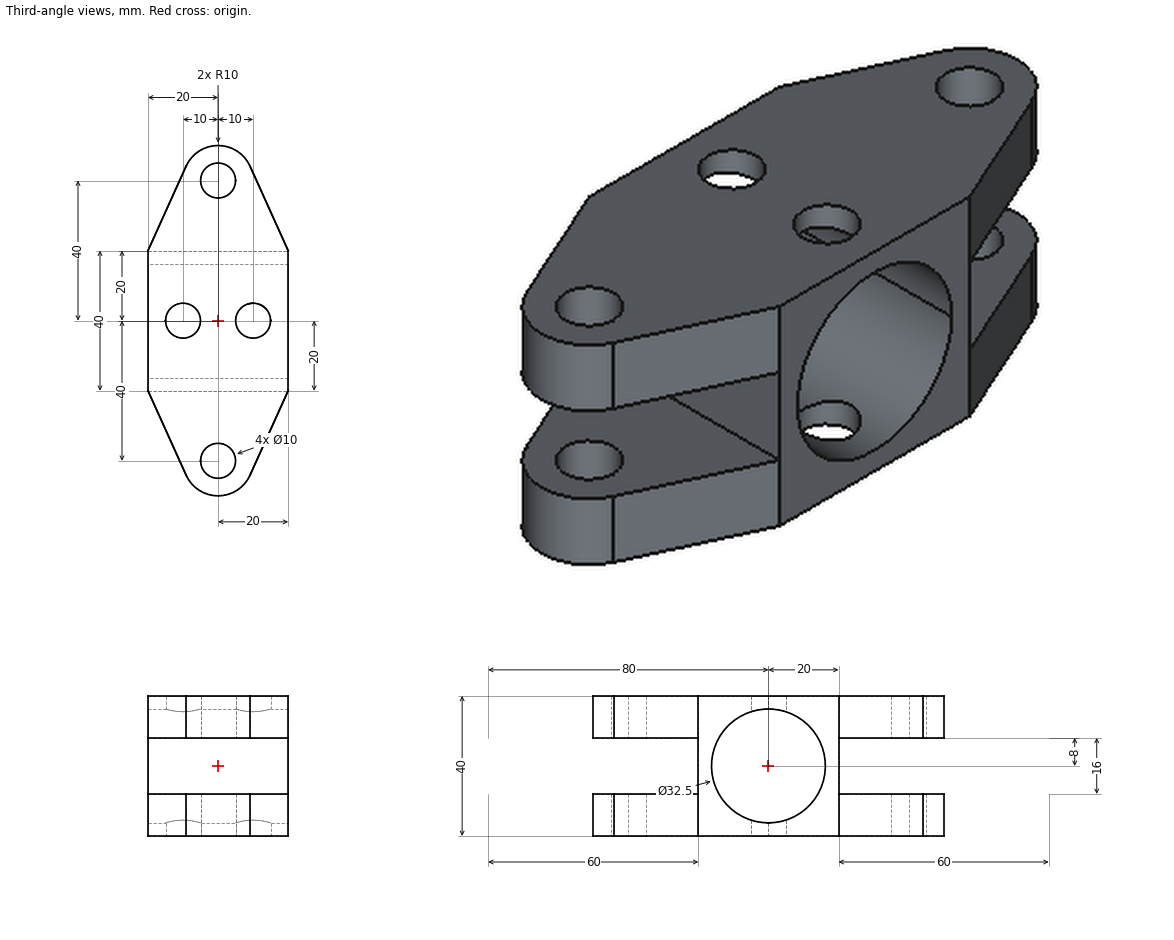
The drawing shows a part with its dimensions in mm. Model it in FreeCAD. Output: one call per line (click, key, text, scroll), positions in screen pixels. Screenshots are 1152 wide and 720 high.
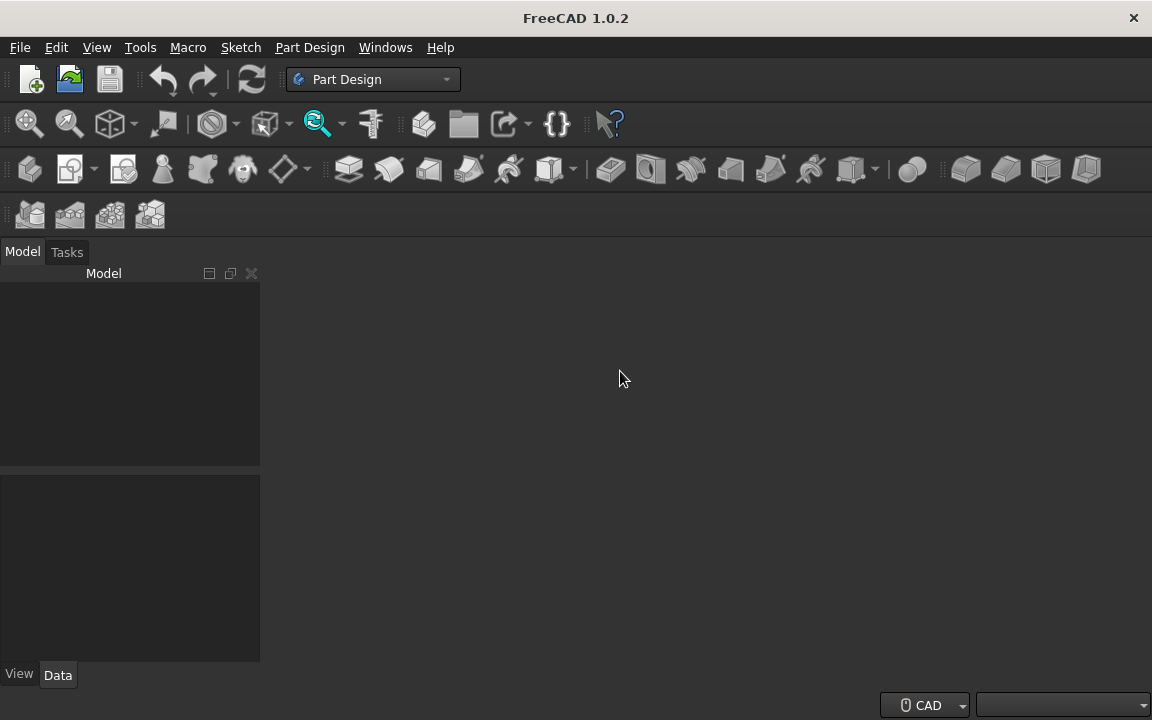
click(30, 80)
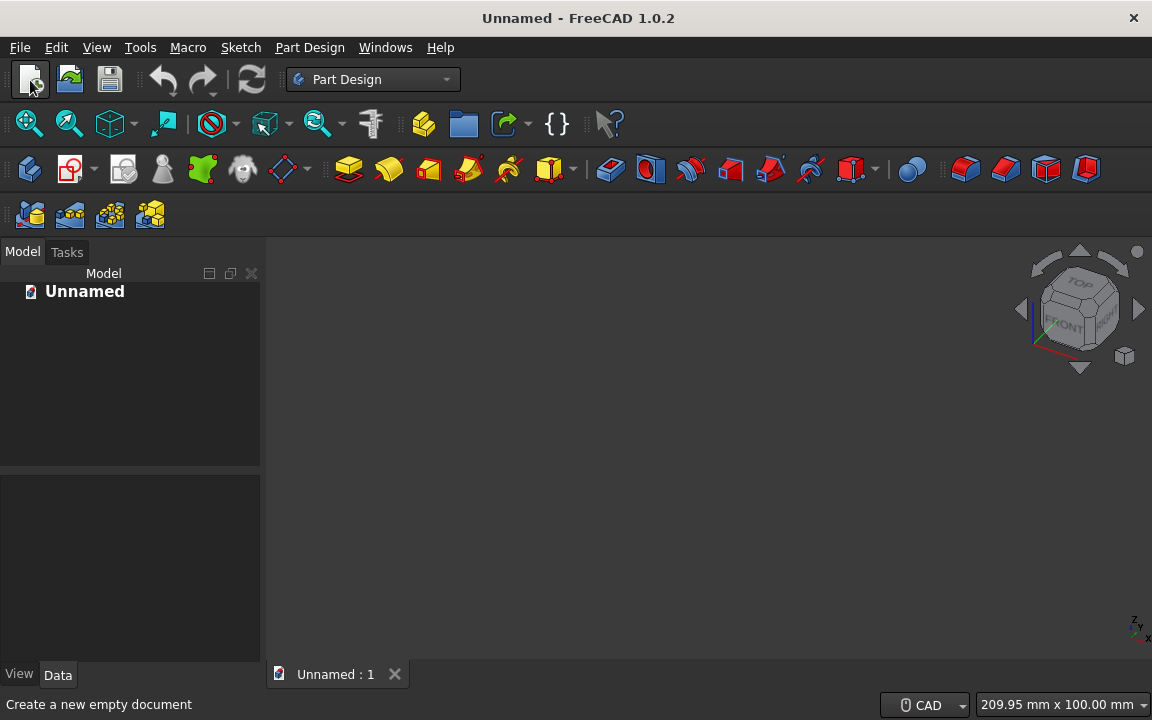
click(70, 170)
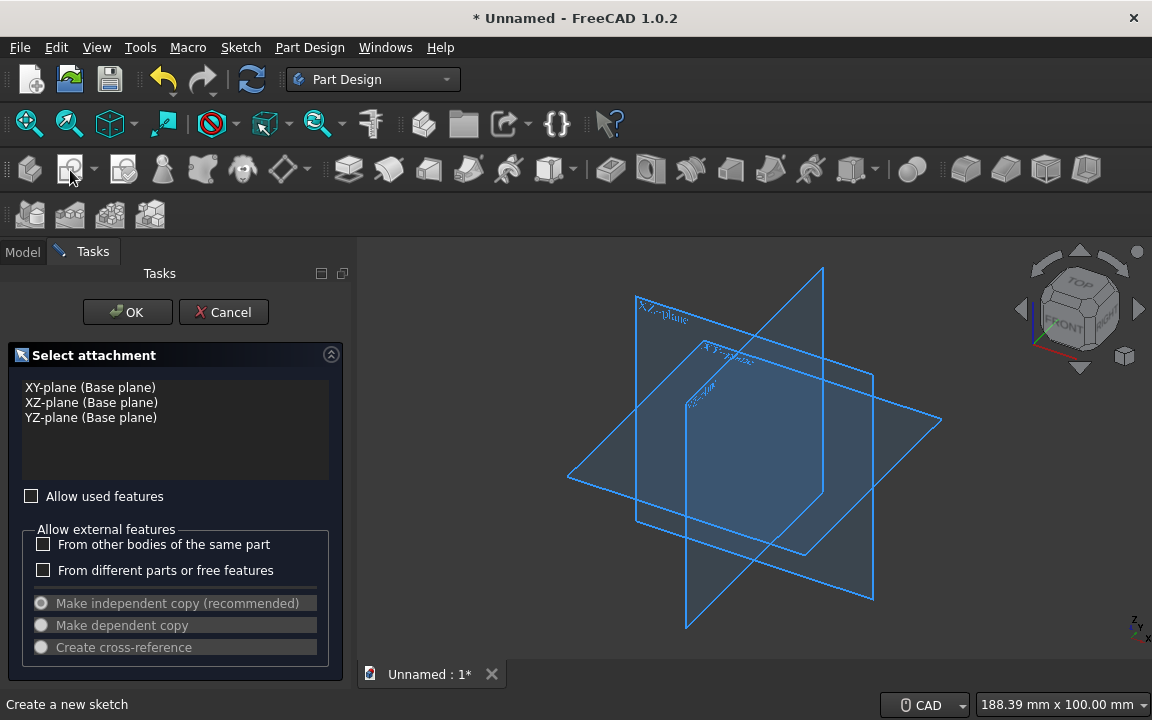
click(82, 388)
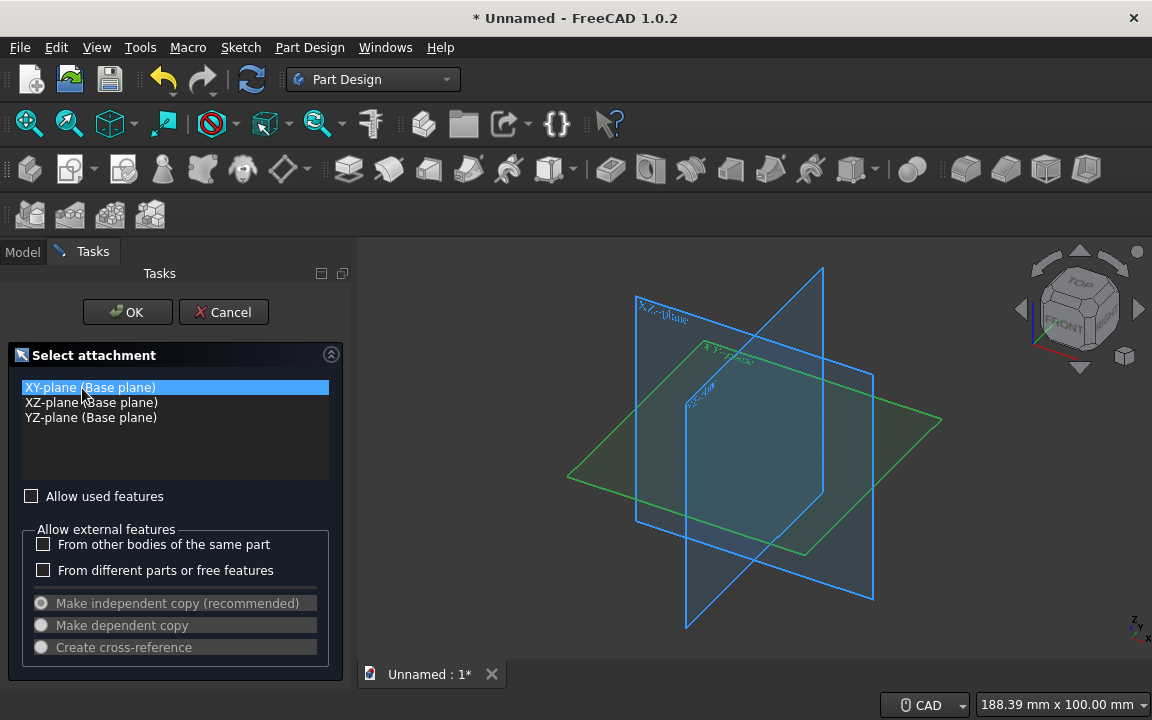
click(128, 312)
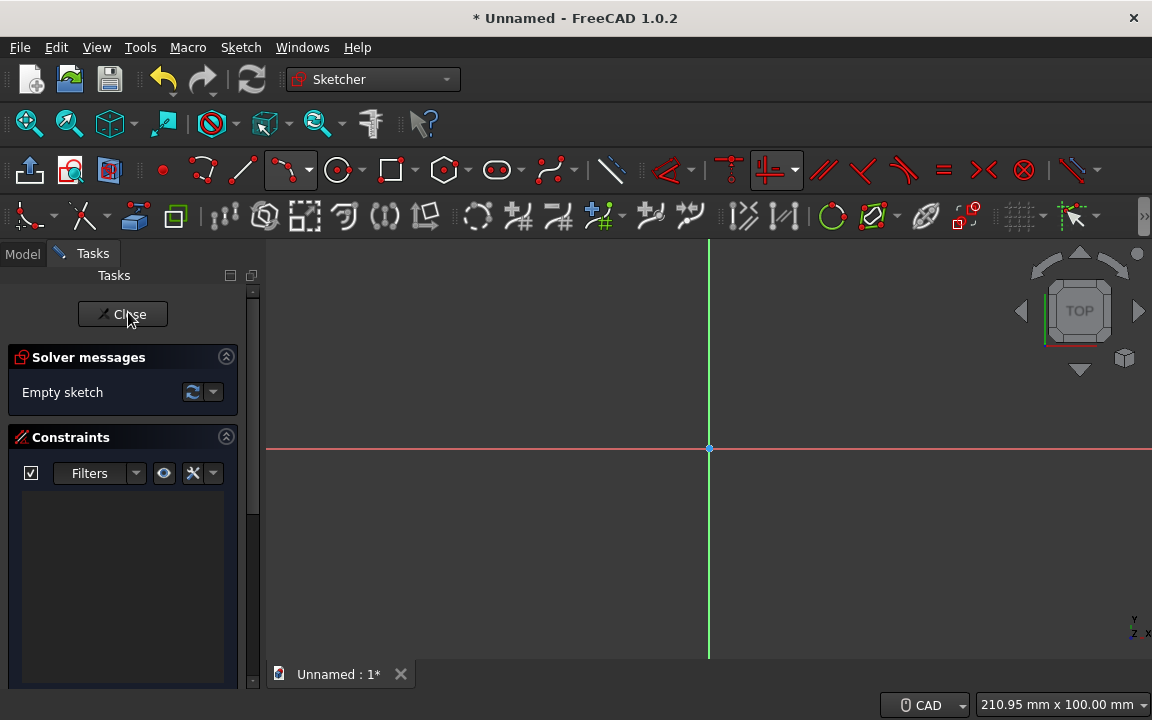
scroll(501, 449, down, 2)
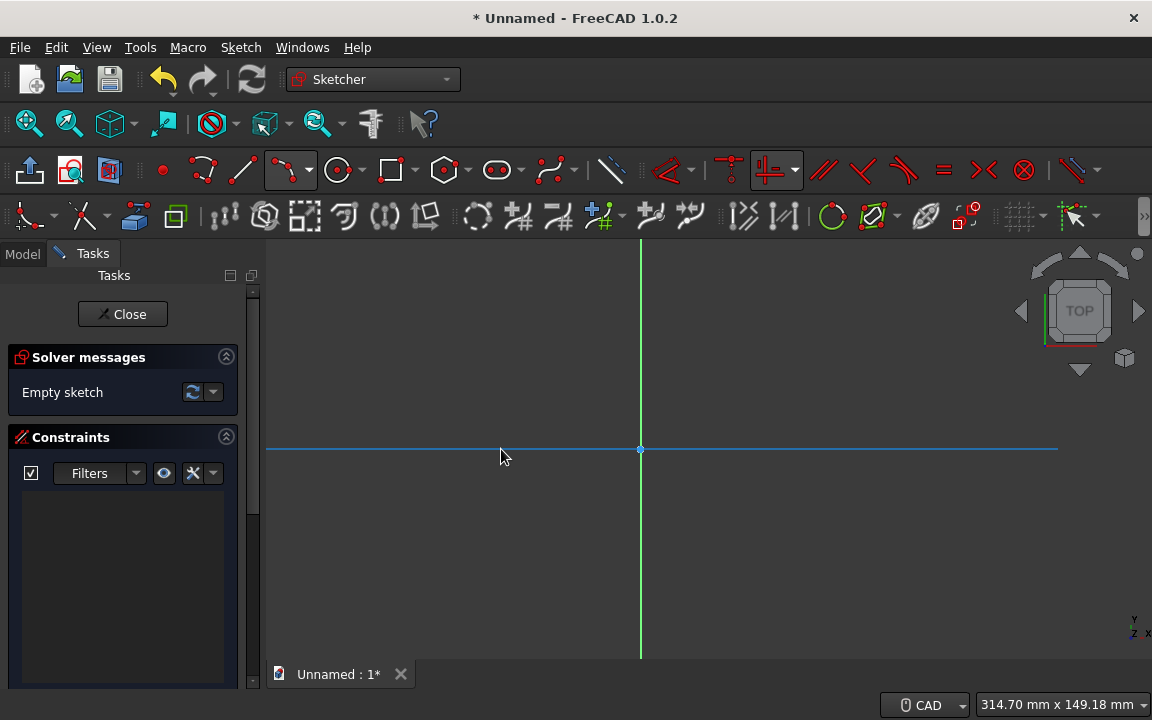
click(204, 170)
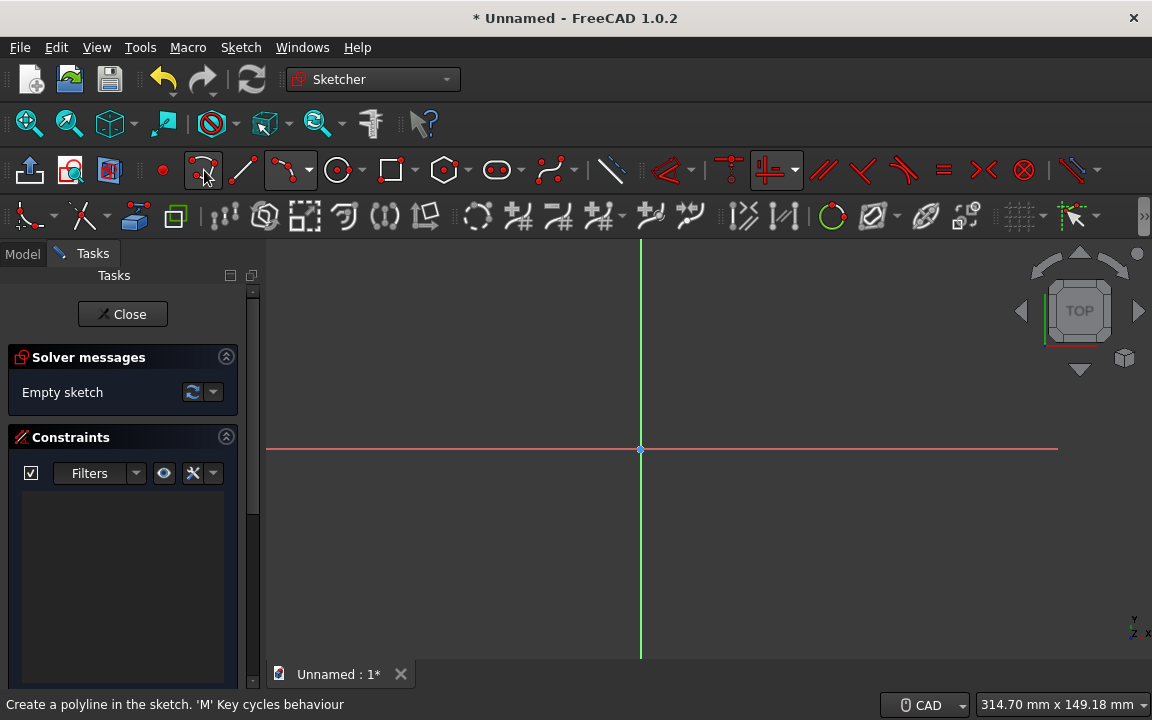
click(615, 325)
click(584, 393)
click(584, 505)
click(615, 573)
right_click(615, 573)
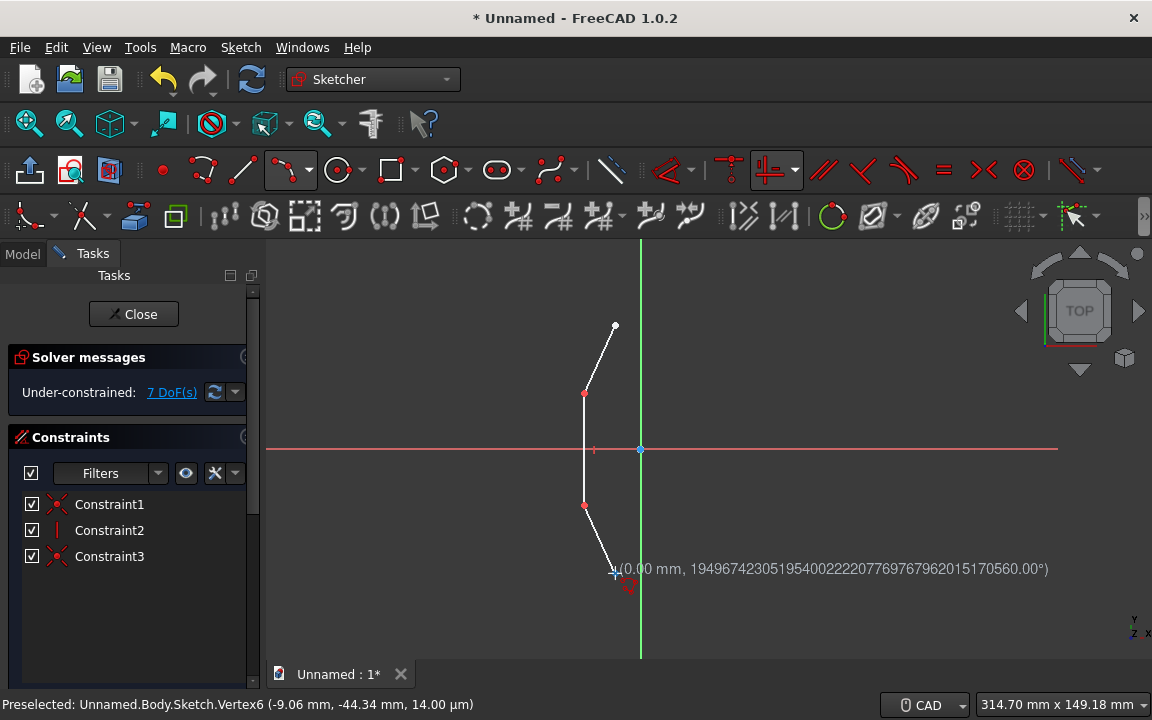
click(666, 573)
click(697, 505)
click(697, 393)
click(666, 325)
right_click(666, 325)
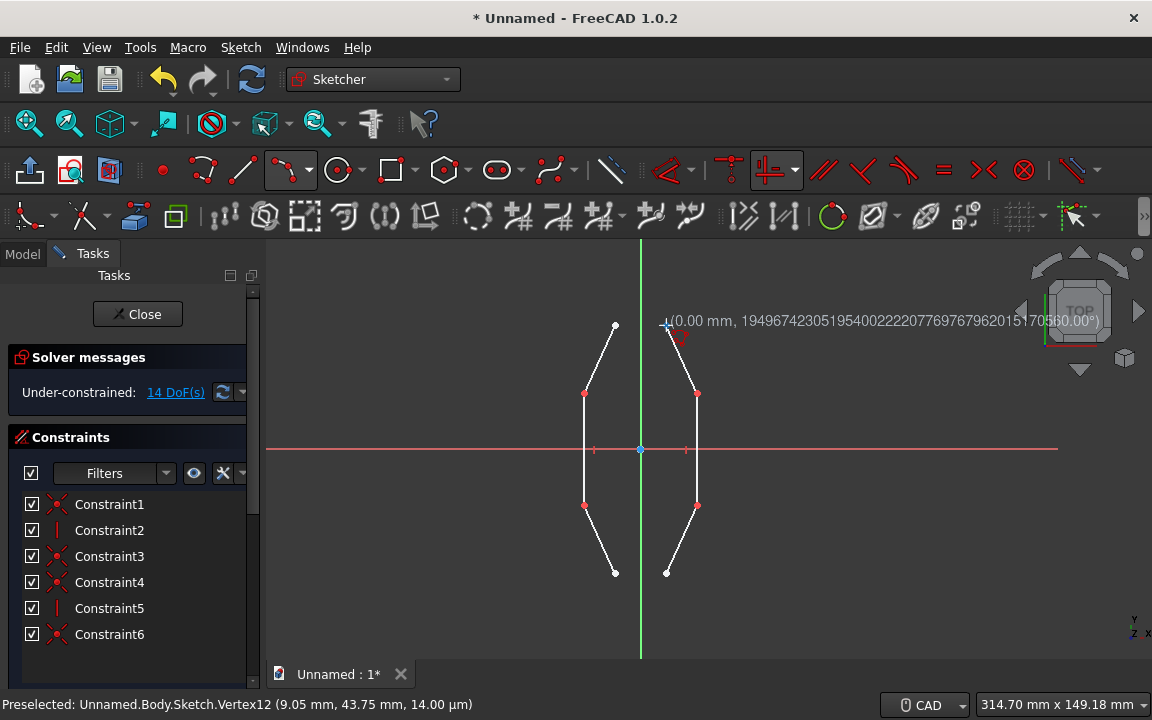
click(284, 170)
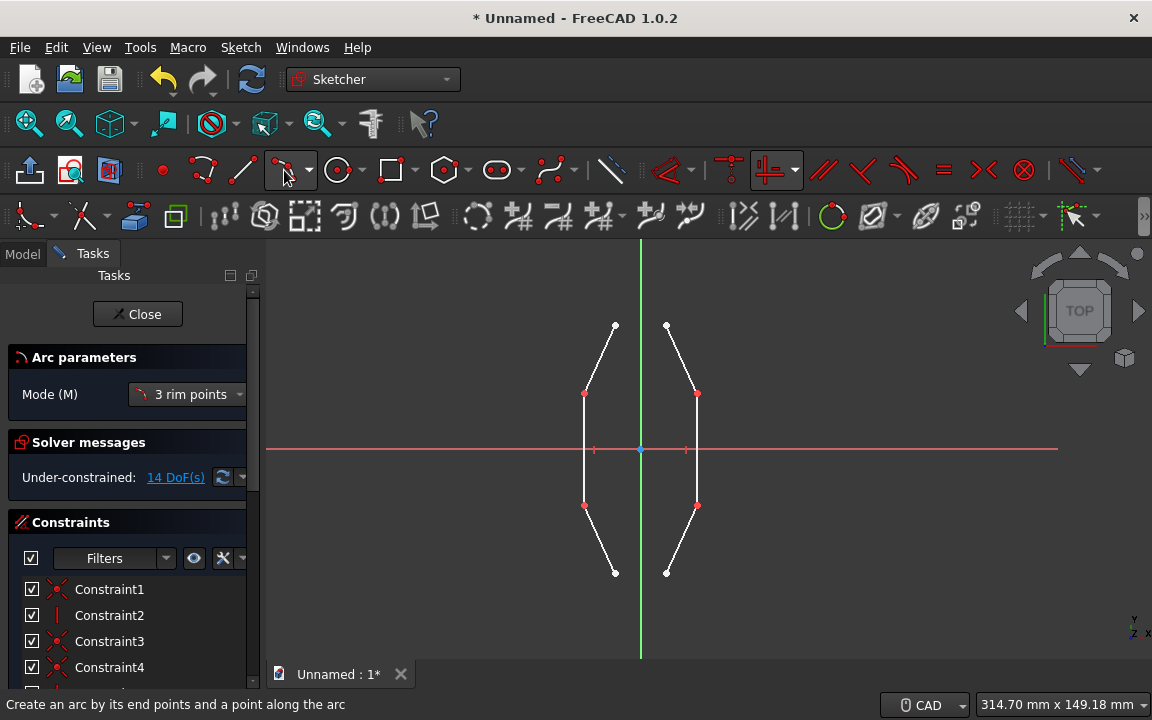
click(615, 574)
click(666, 574)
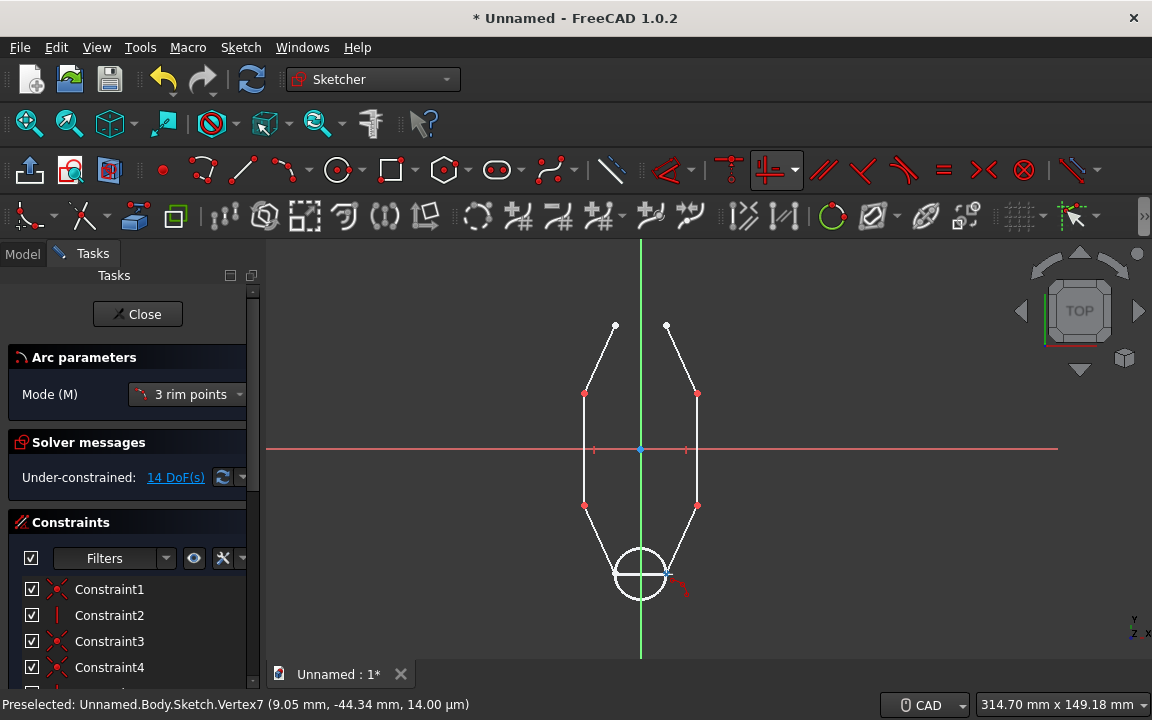
scroll(653, 587, up, 2)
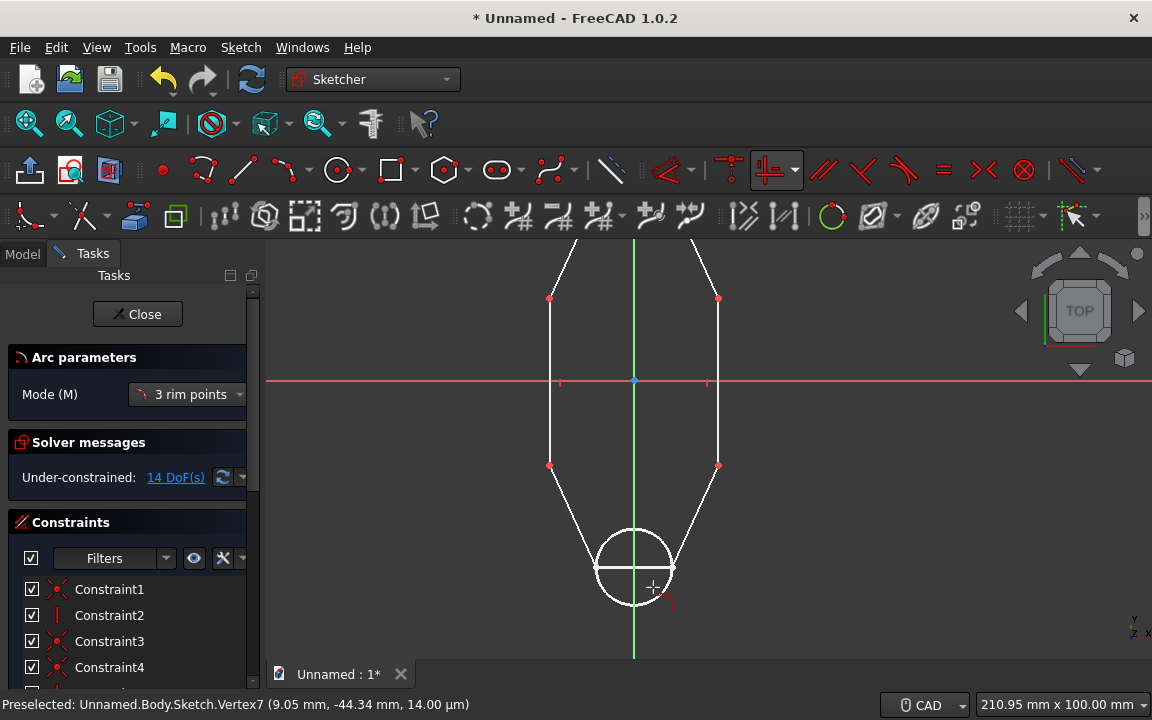
click(653, 587)